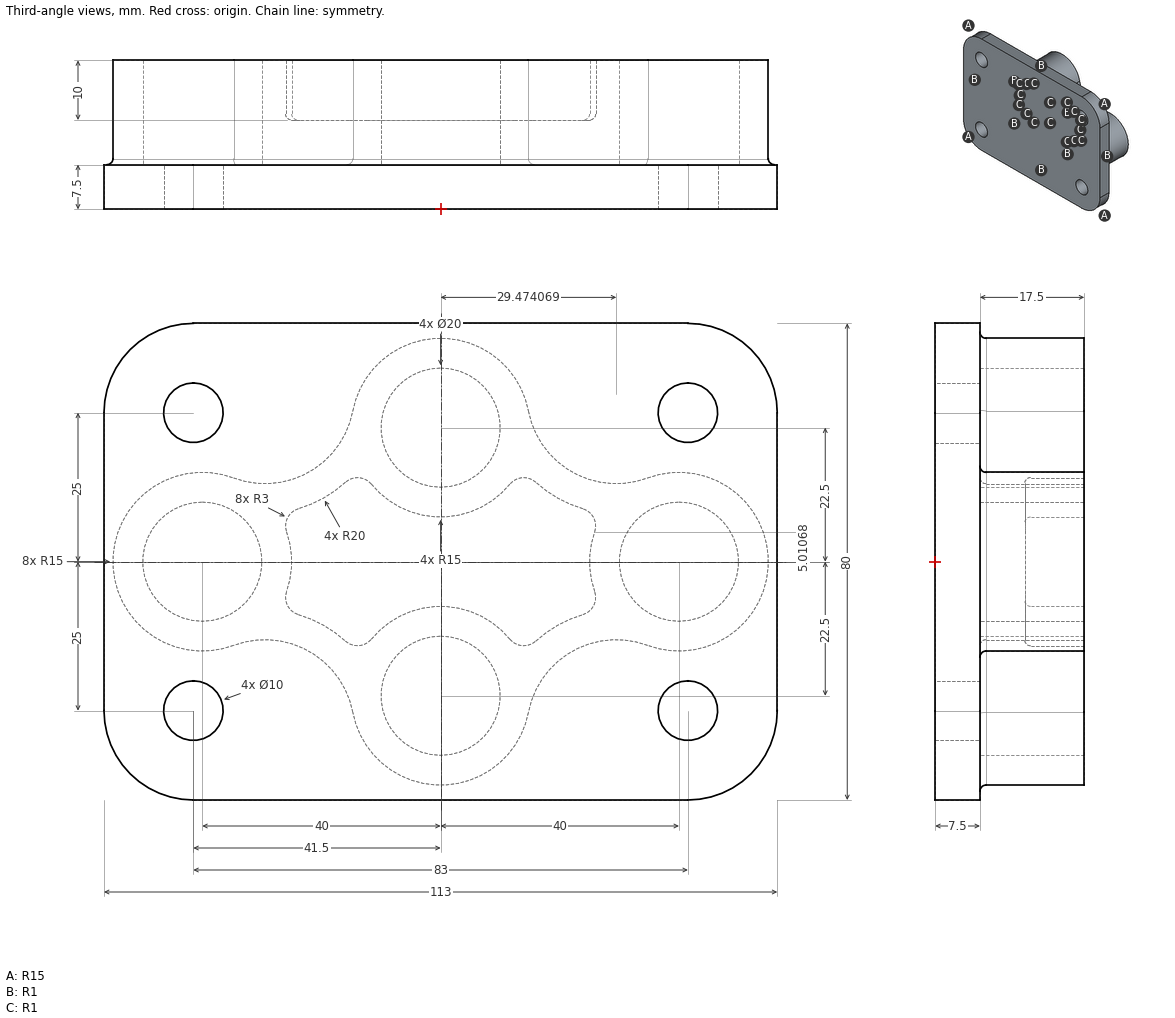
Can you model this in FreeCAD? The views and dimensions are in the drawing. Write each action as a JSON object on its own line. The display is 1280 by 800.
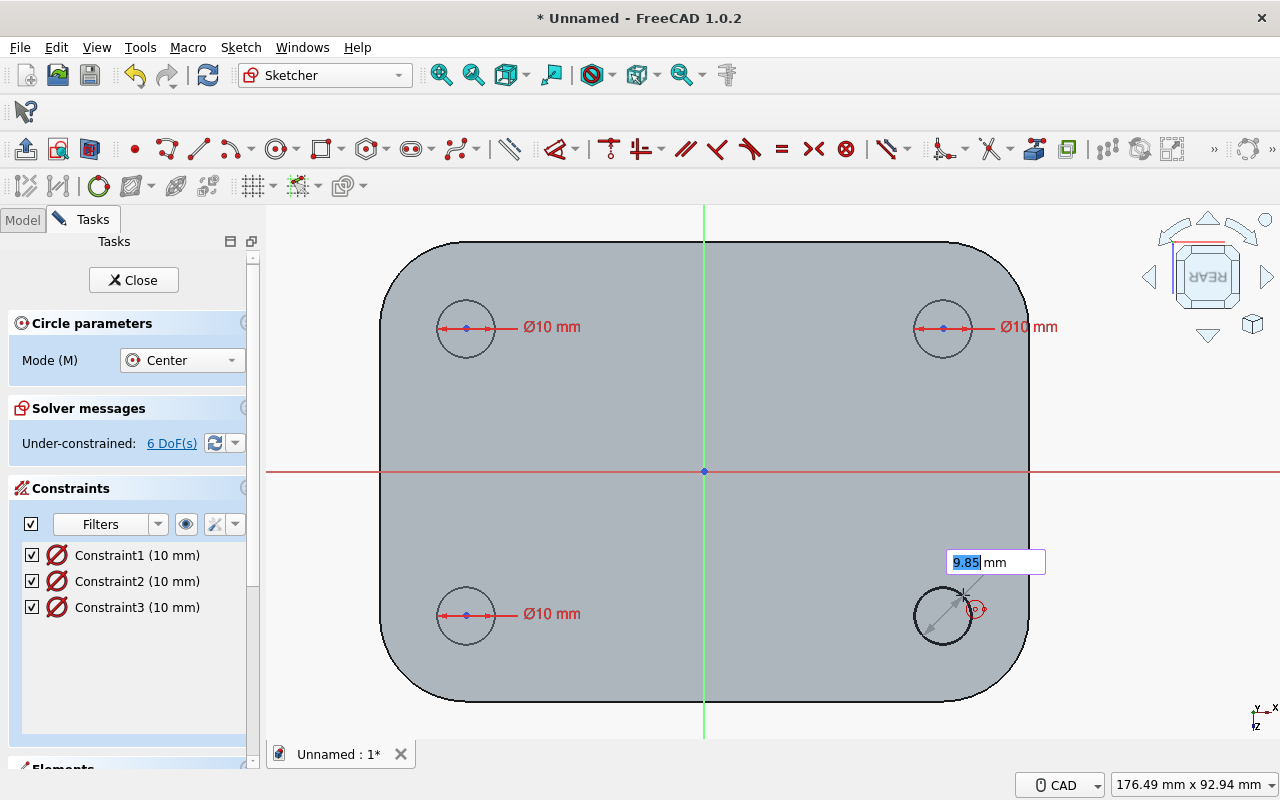
{"action": "type", "text": "10"}
{"action": "key", "text": "Return"}
{"action": "key", "text": "Escape"}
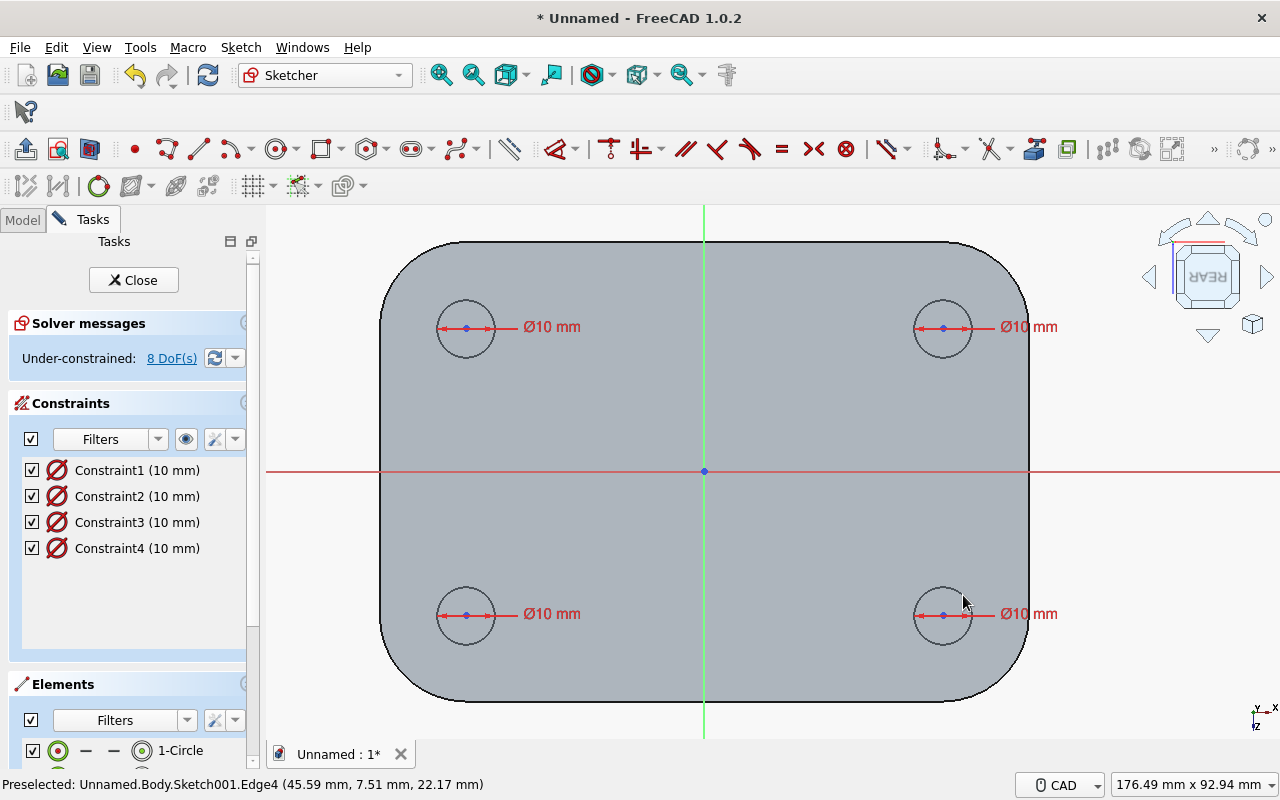
{"action": "left_click", "coordinate": [466, 329]}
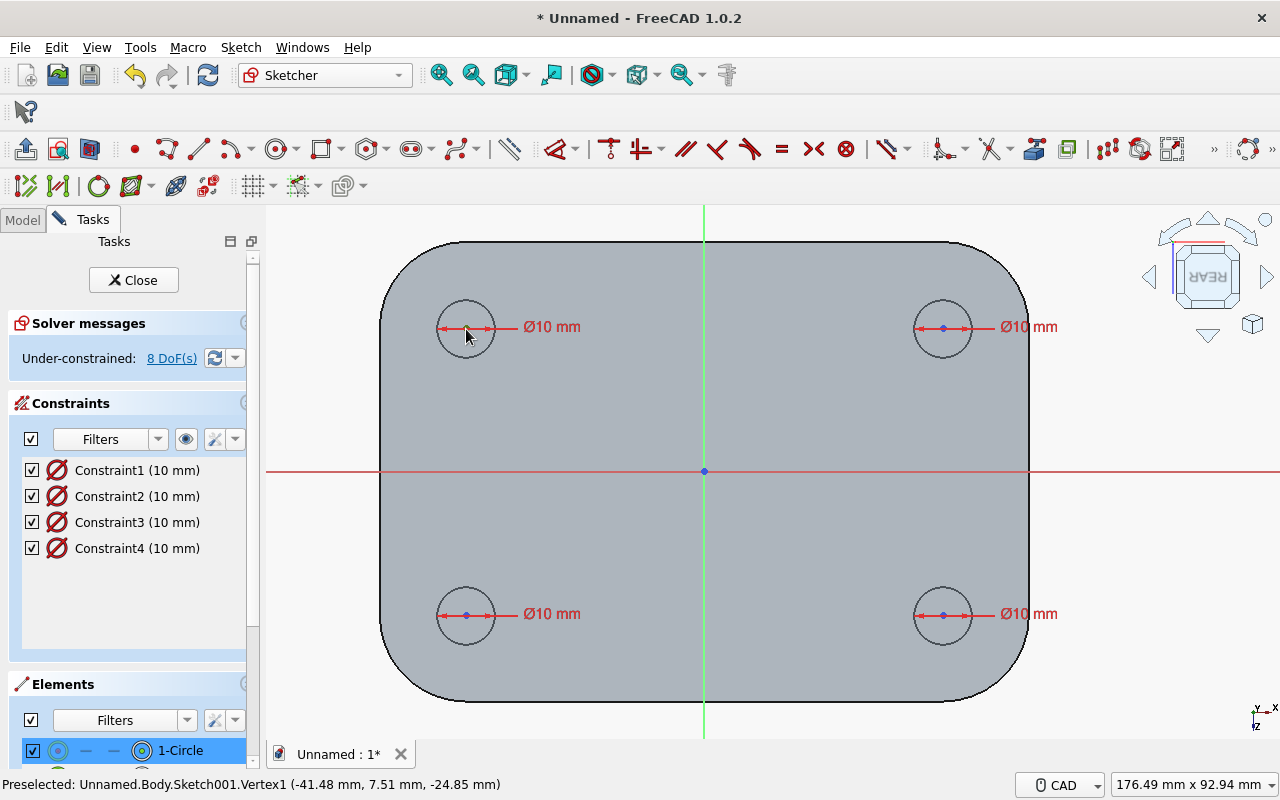
{"action": "left_click", "coordinate": [943, 329]}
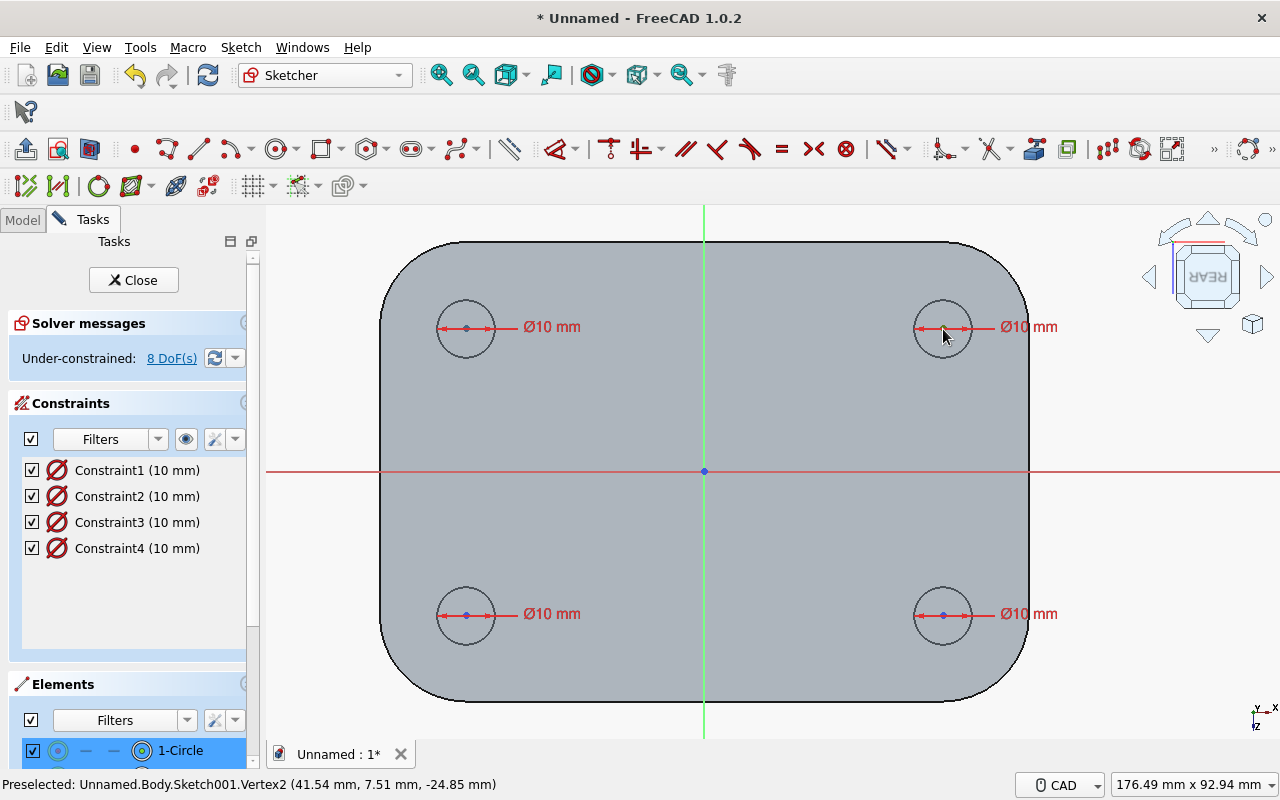
{"action": "key", "text": "h"}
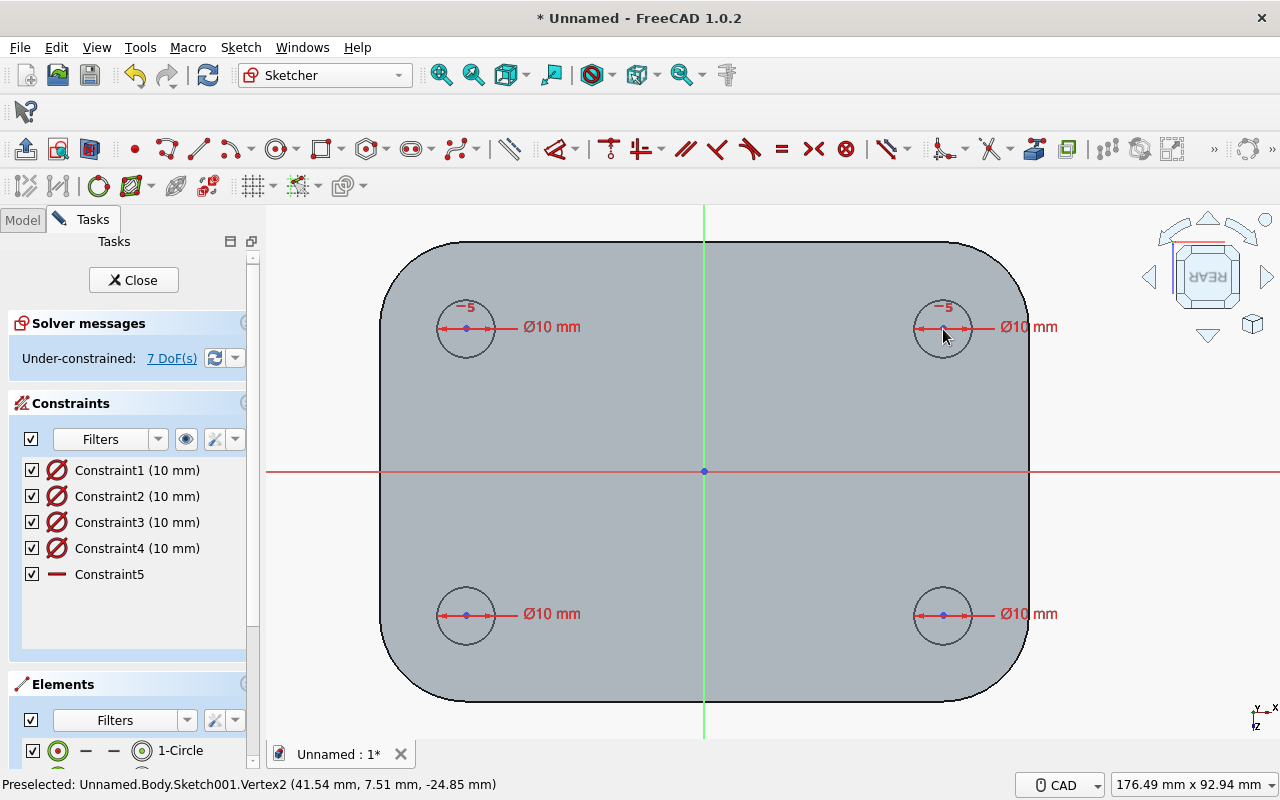
{"action": "left_click", "coordinate": [466, 329]}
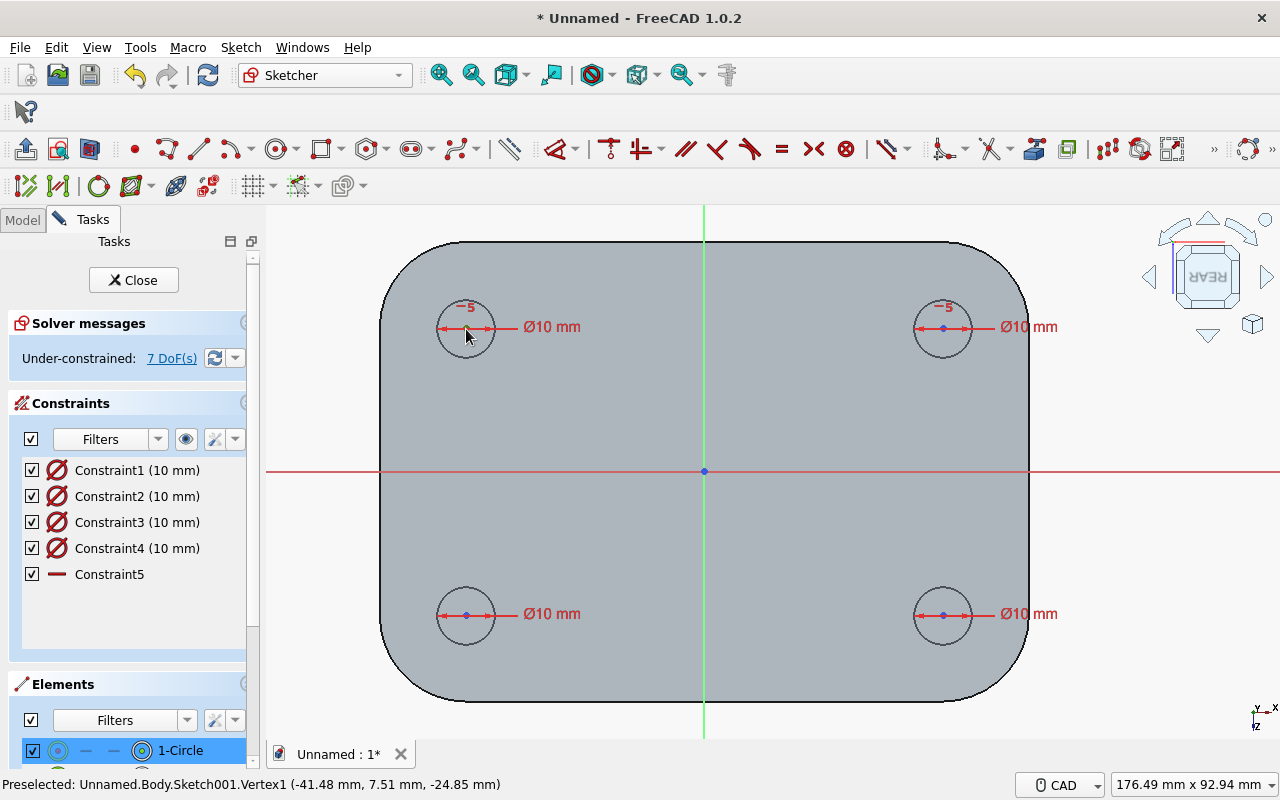
{"action": "left_click", "coordinate": [466, 616]}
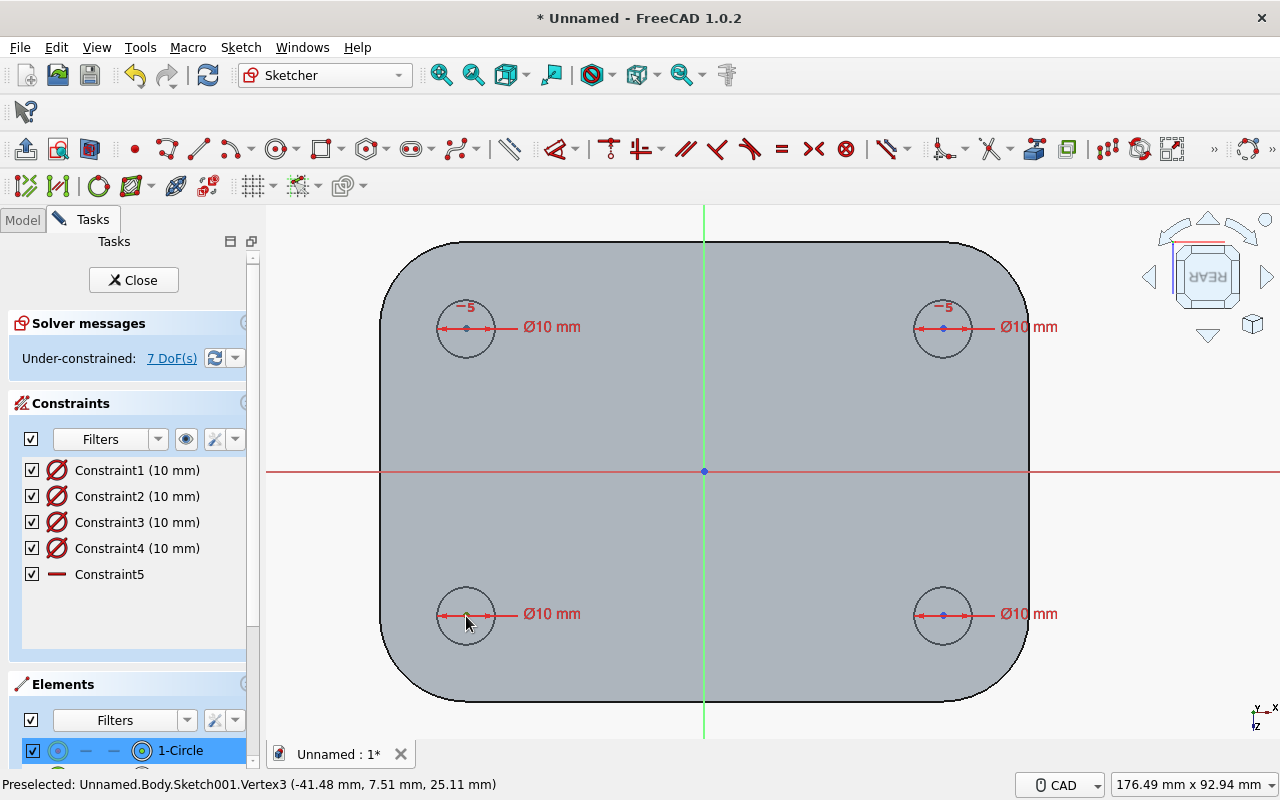
{"action": "key", "text": "v"}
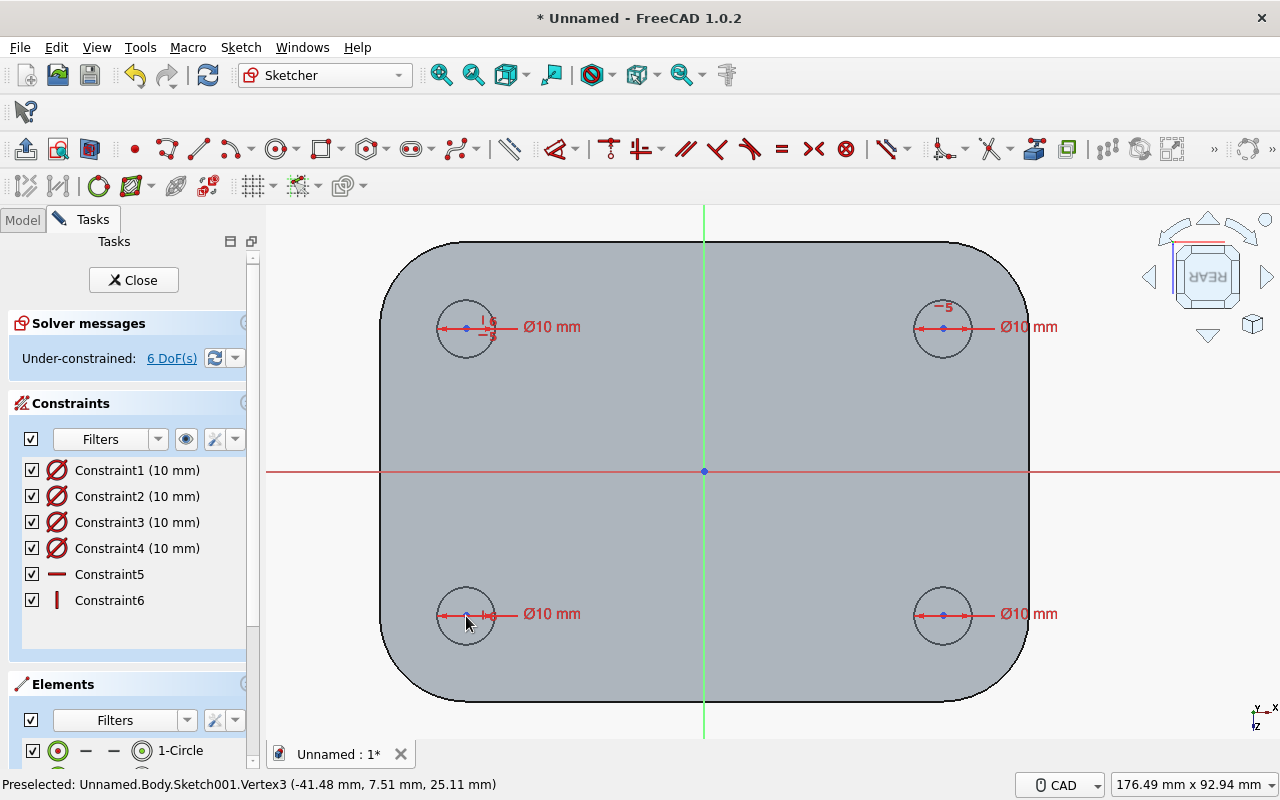
{"action": "left_click", "coordinate": [943, 329]}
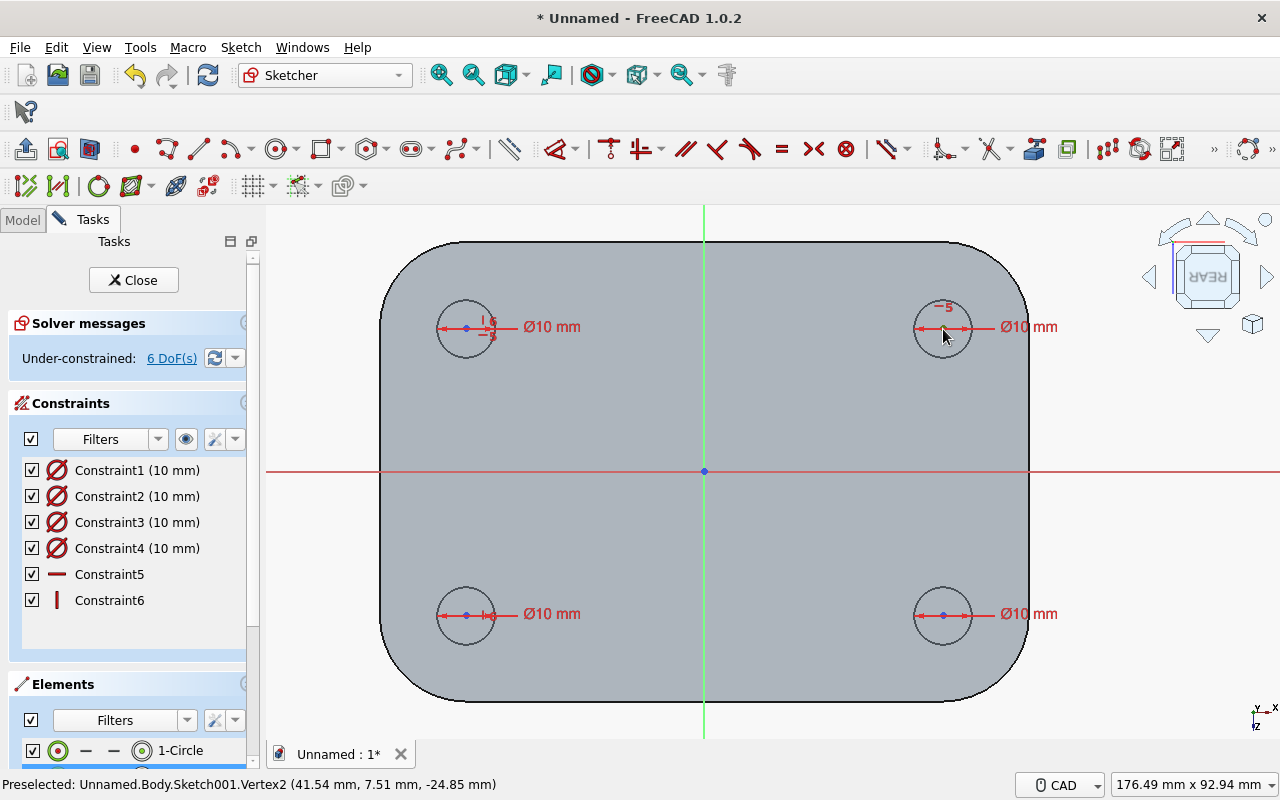
{"action": "left_click", "coordinate": [943, 616]}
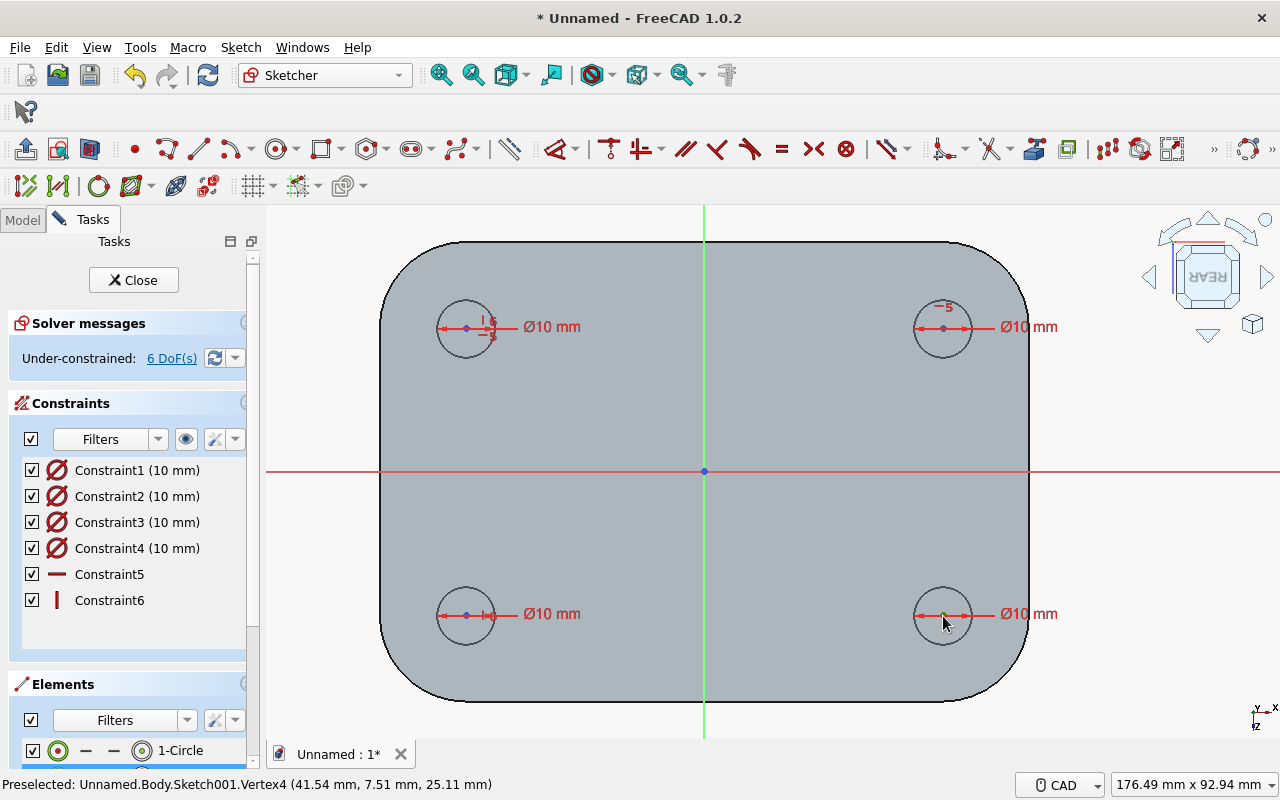
{"action": "key", "text": "v"}